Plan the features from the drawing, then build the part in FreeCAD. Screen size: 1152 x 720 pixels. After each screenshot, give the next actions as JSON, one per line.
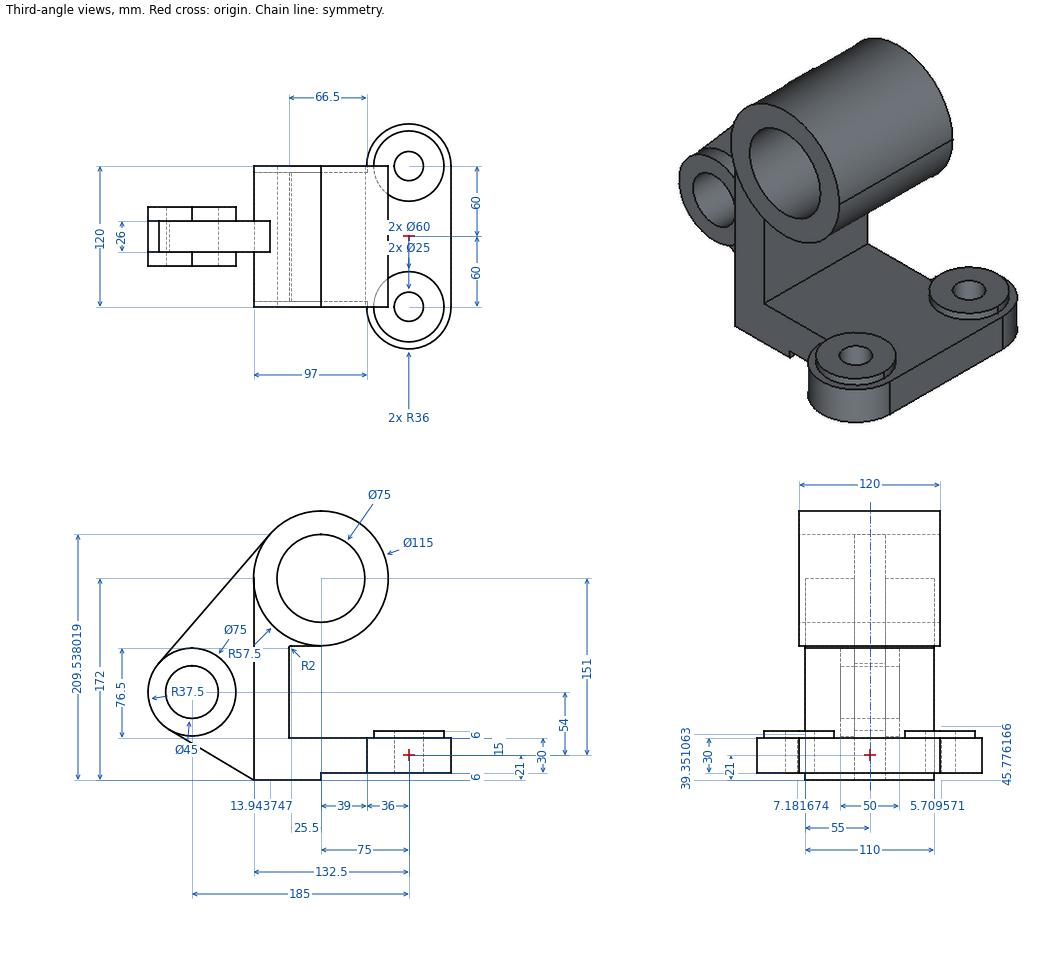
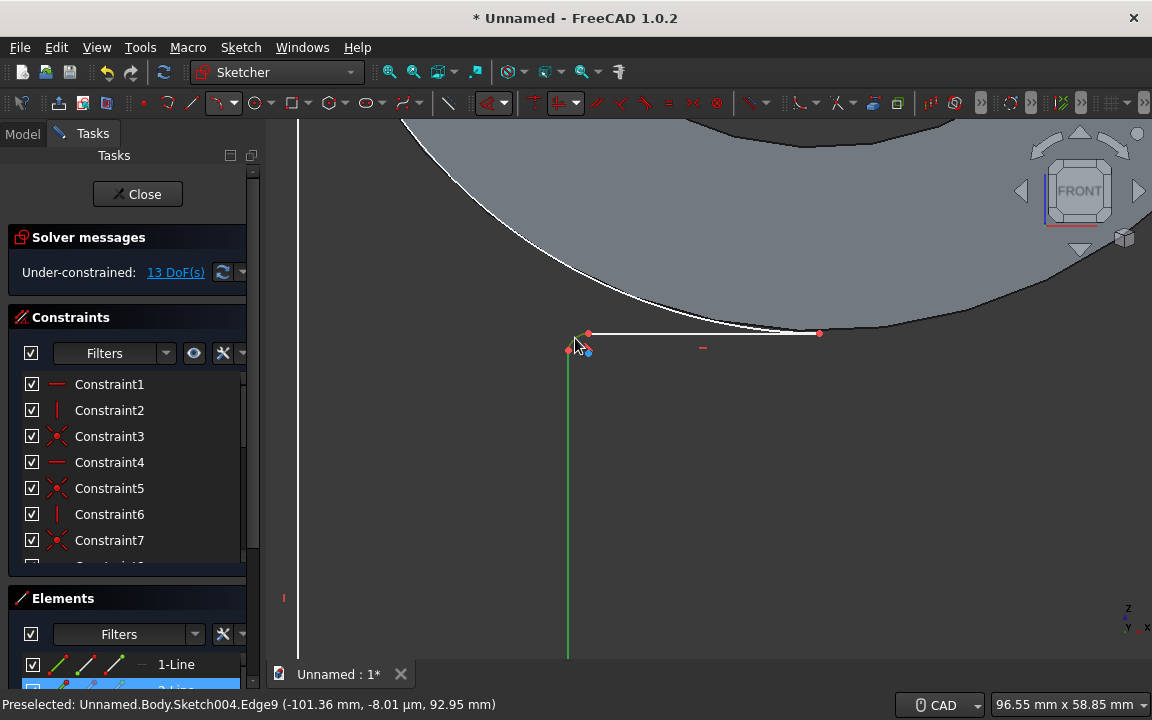
{"action": "left_click", "coordinate": [646, 104]}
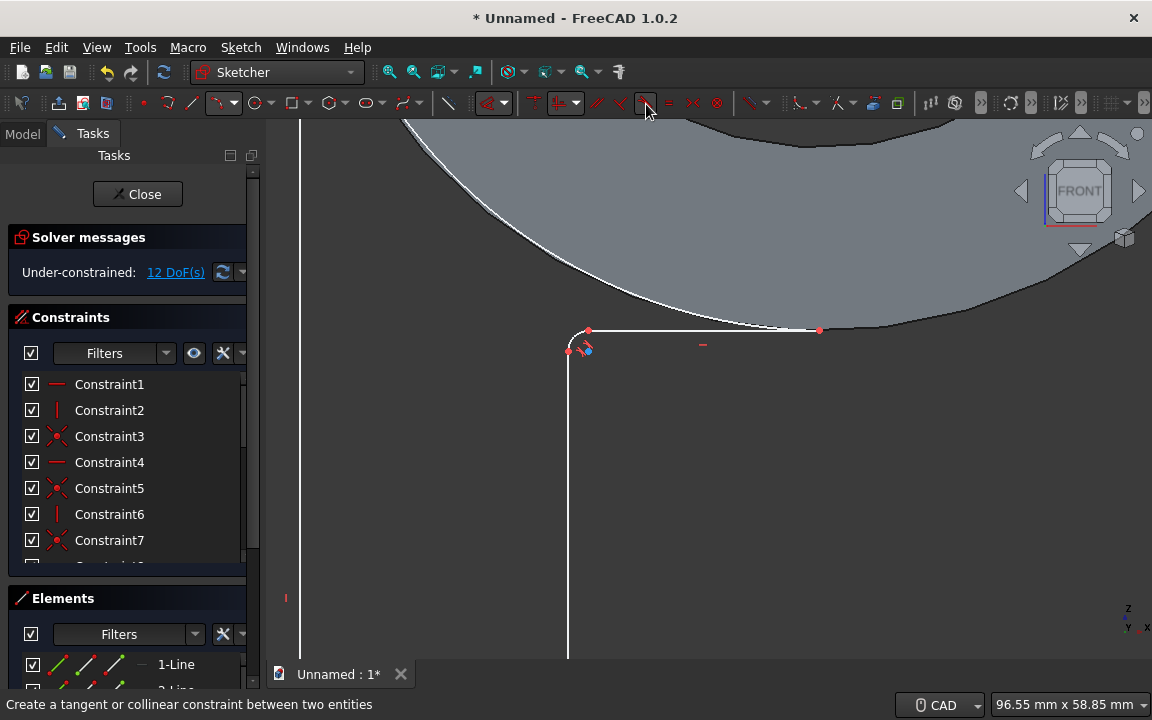
{"action": "scroll", "coordinate": [579, 333], "scroll_direction": "up", "scroll_amount": 4}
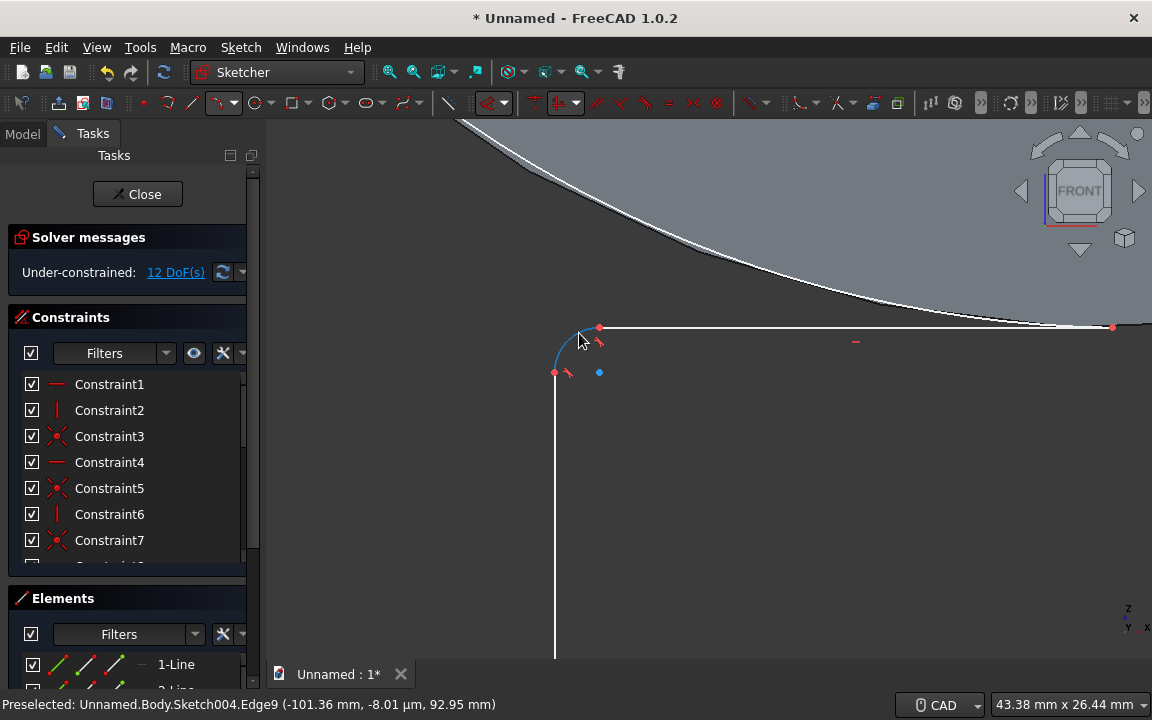
{"action": "left_click", "coordinate": [579, 333]}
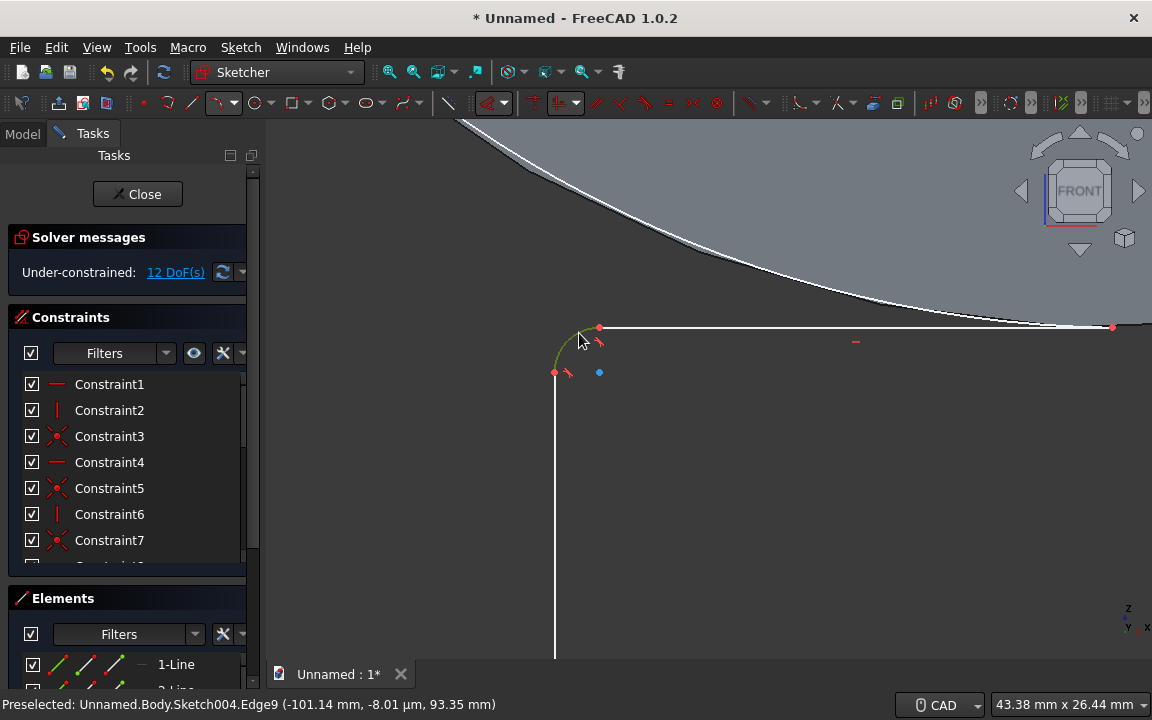
{"action": "key", "text": "k r"}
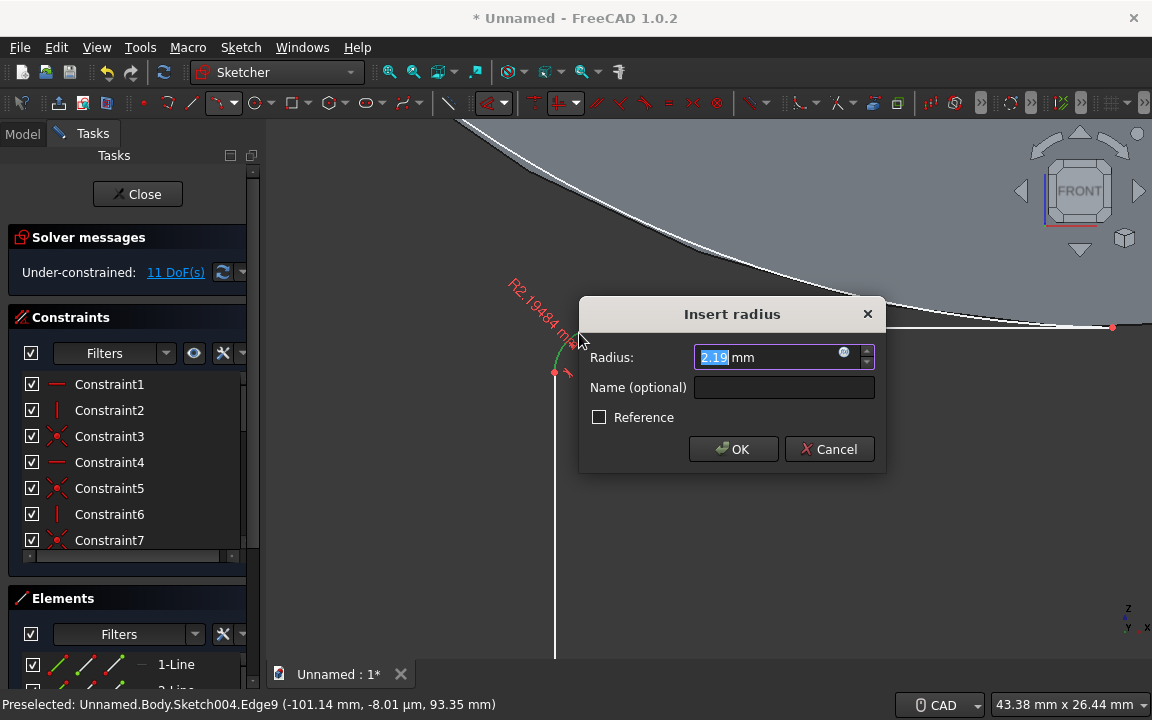
{"action": "type", "text": "2"}
{"action": "key", "text": "Return"}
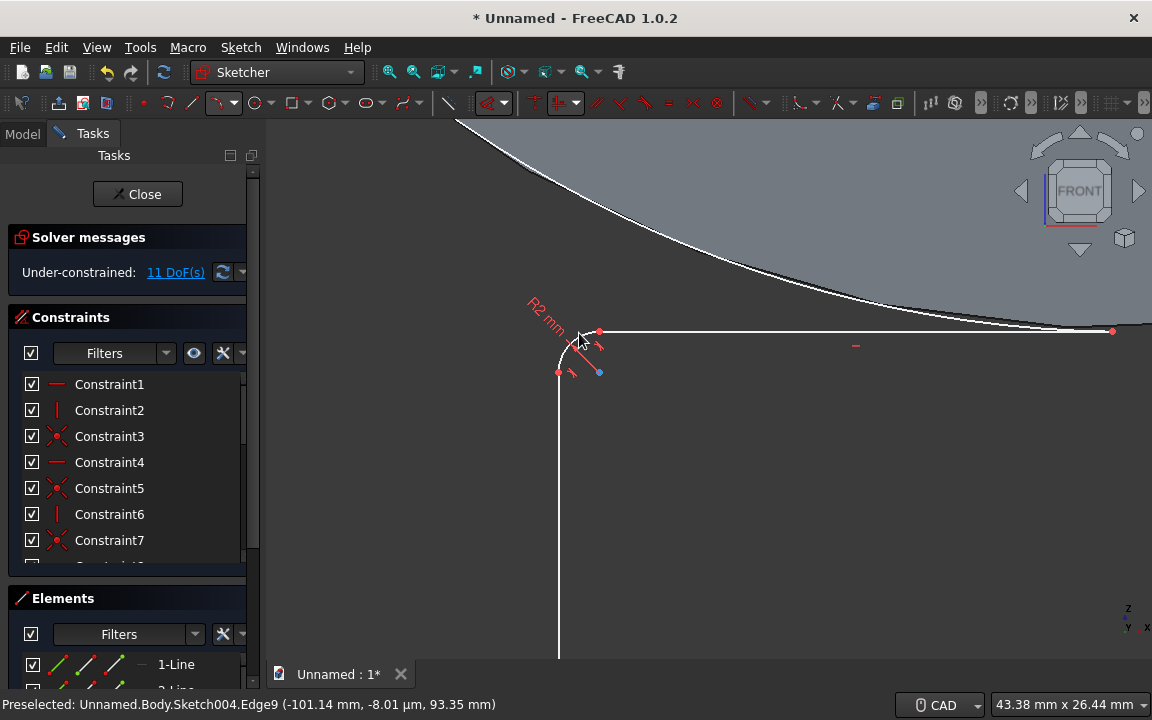
{"action": "scroll", "coordinate": [575, 337], "scroll_direction": "down", "scroll_amount": 12}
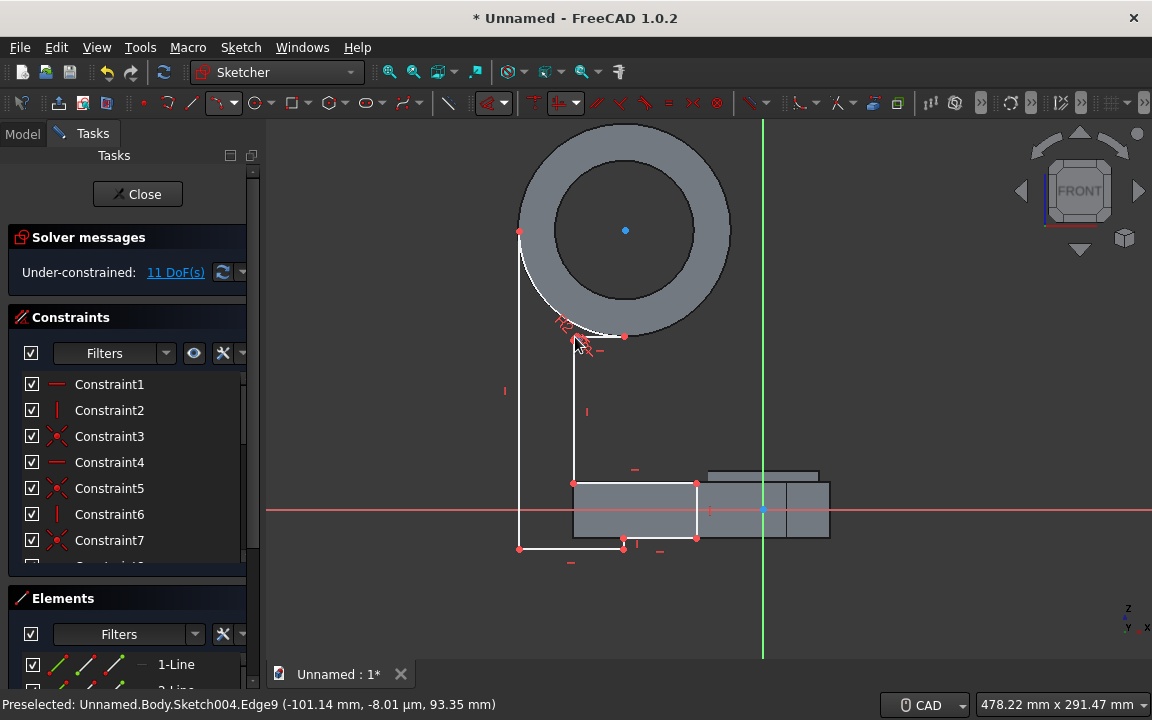
{"action": "left_click", "coordinate": [577, 325]}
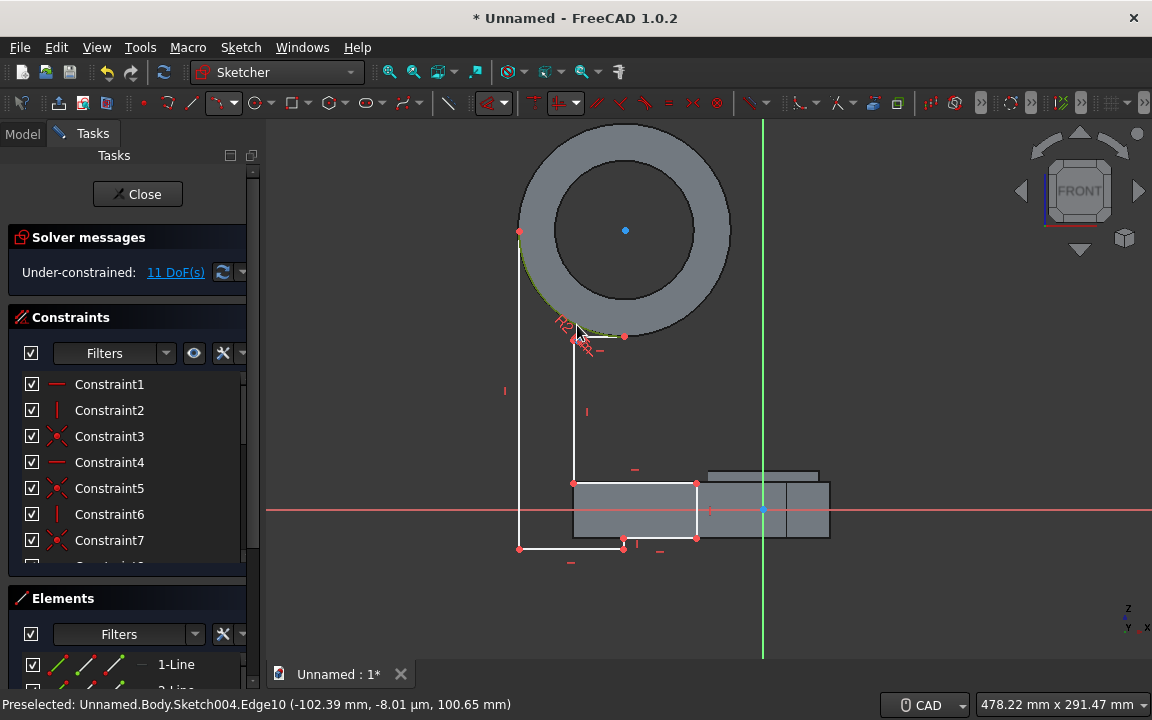
{"action": "key", "text": "k r"}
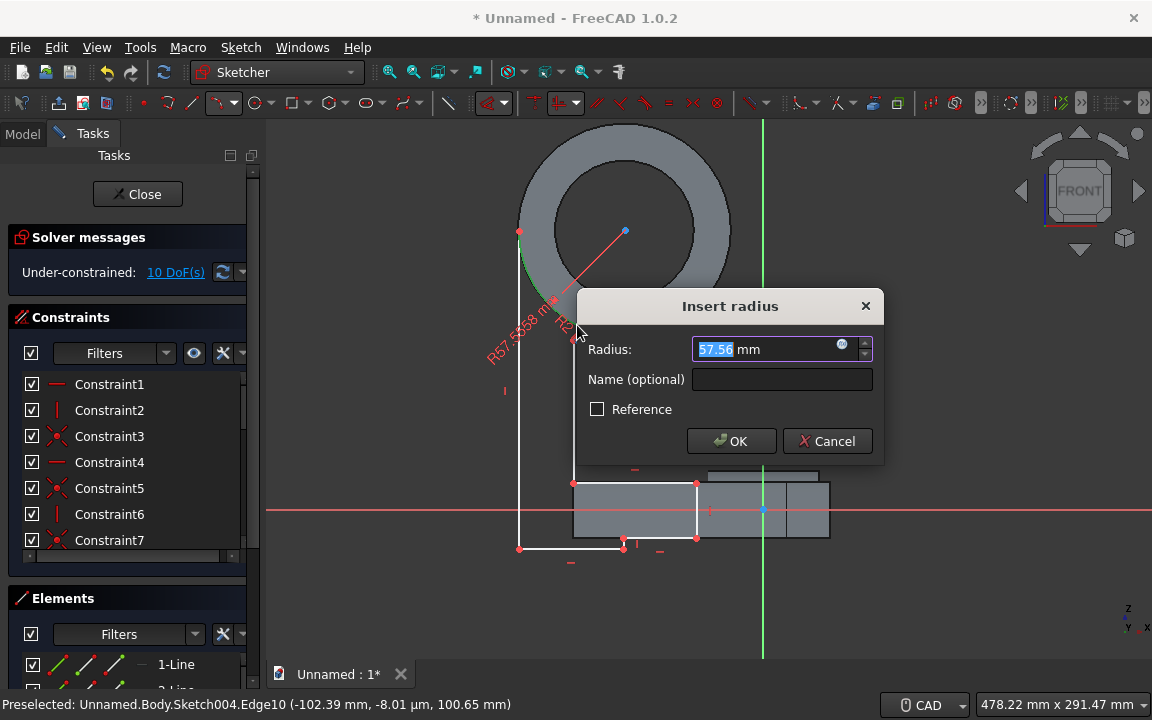
{"action": "type", "text": "57.5"}
{"action": "key", "text": "Return"}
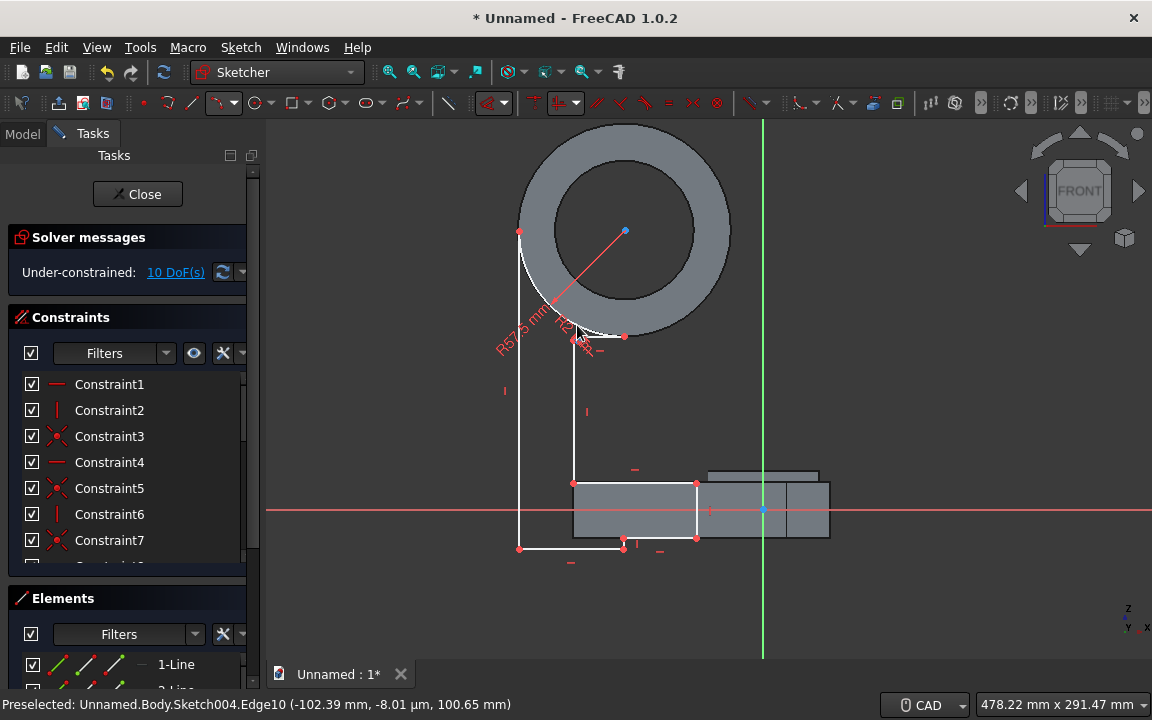
{"action": "scroll", "coordinate": [624, 544], "scroll_direction": "up", "scroll_amount": 7}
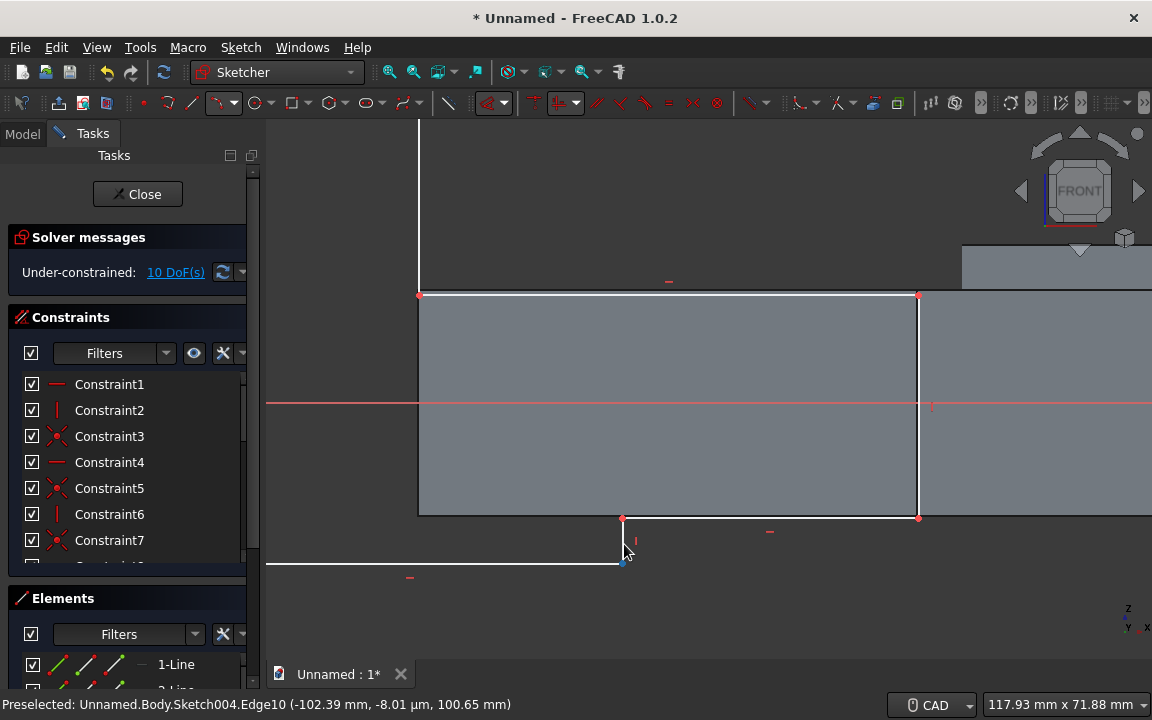
{"action": "left_click", "coordinate": [623, 541]}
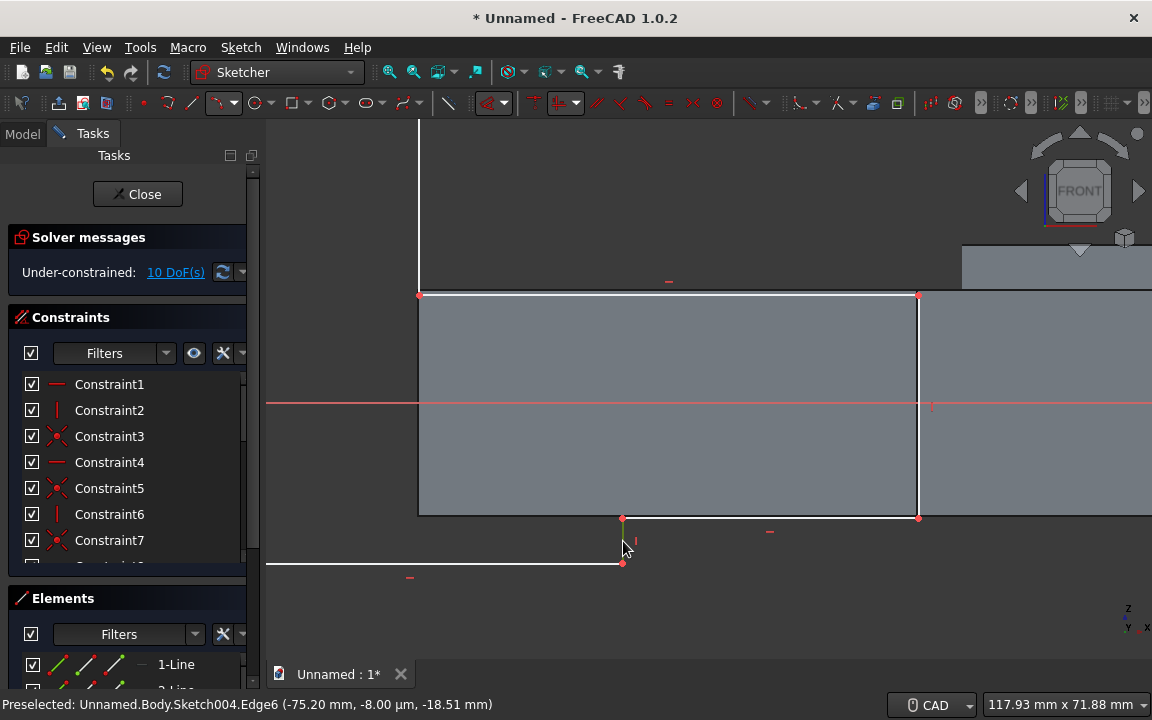
{"action": "left_click", "coordinate": [506, 104]}